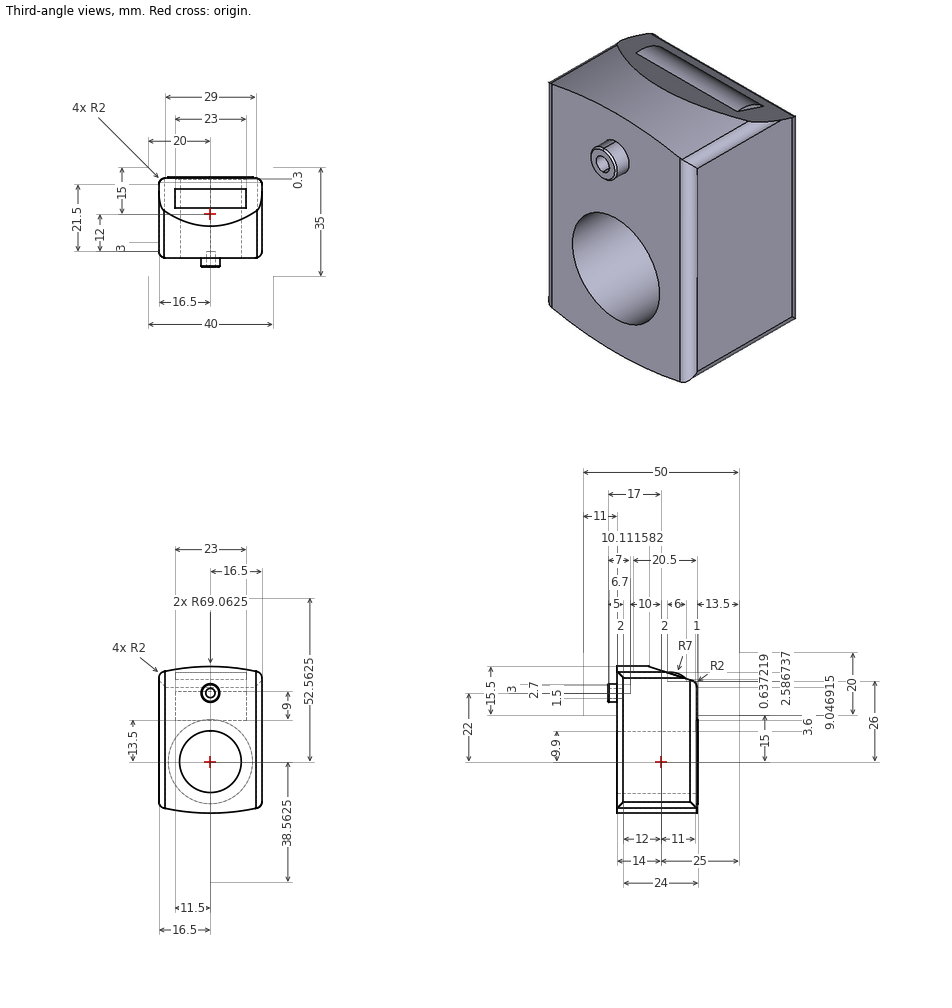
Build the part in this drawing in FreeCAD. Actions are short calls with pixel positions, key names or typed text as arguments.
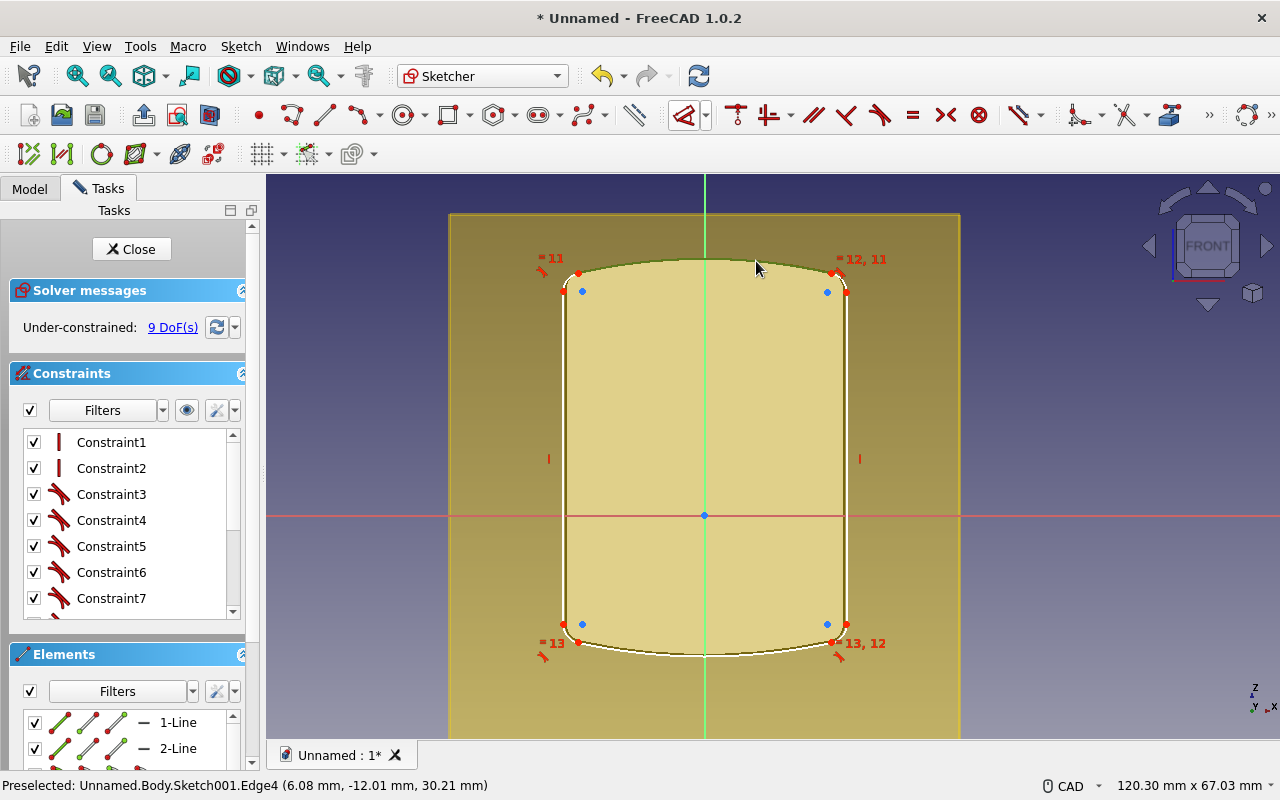
click(654, 654)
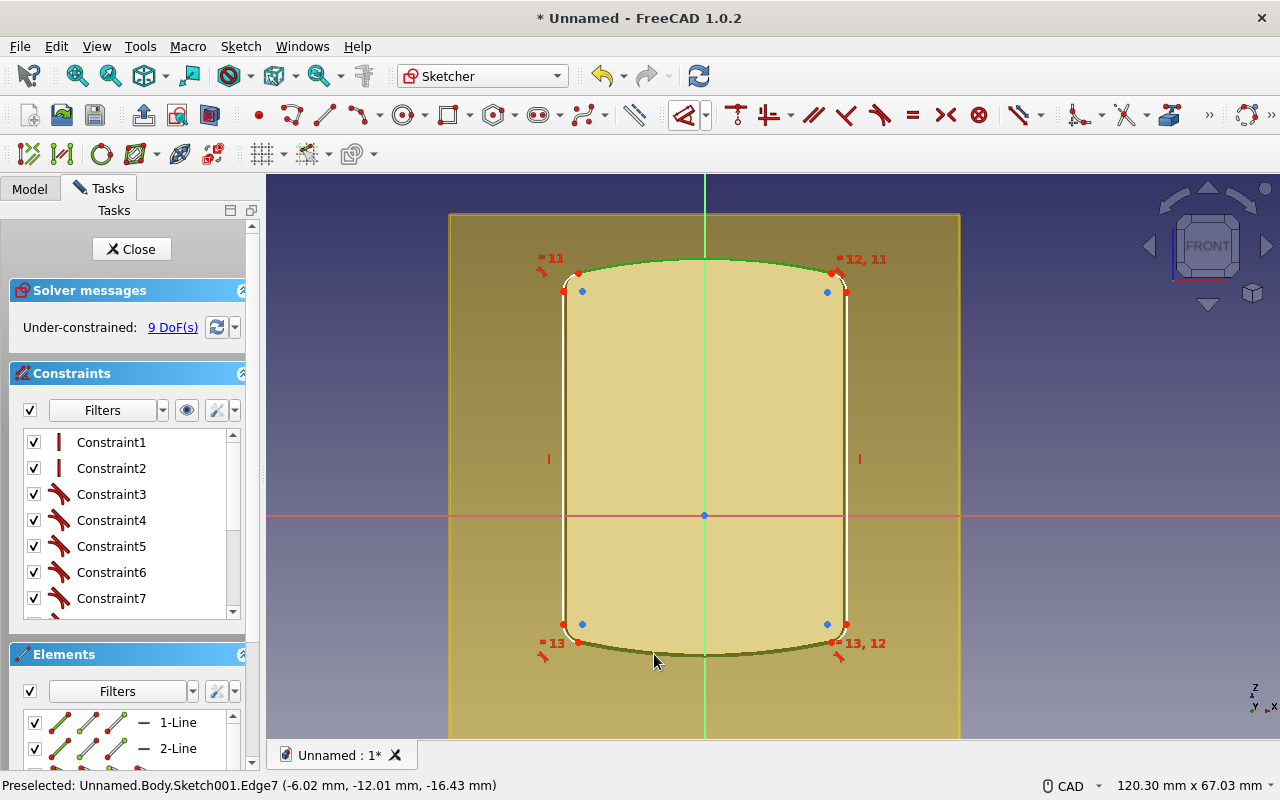
click(913, 116)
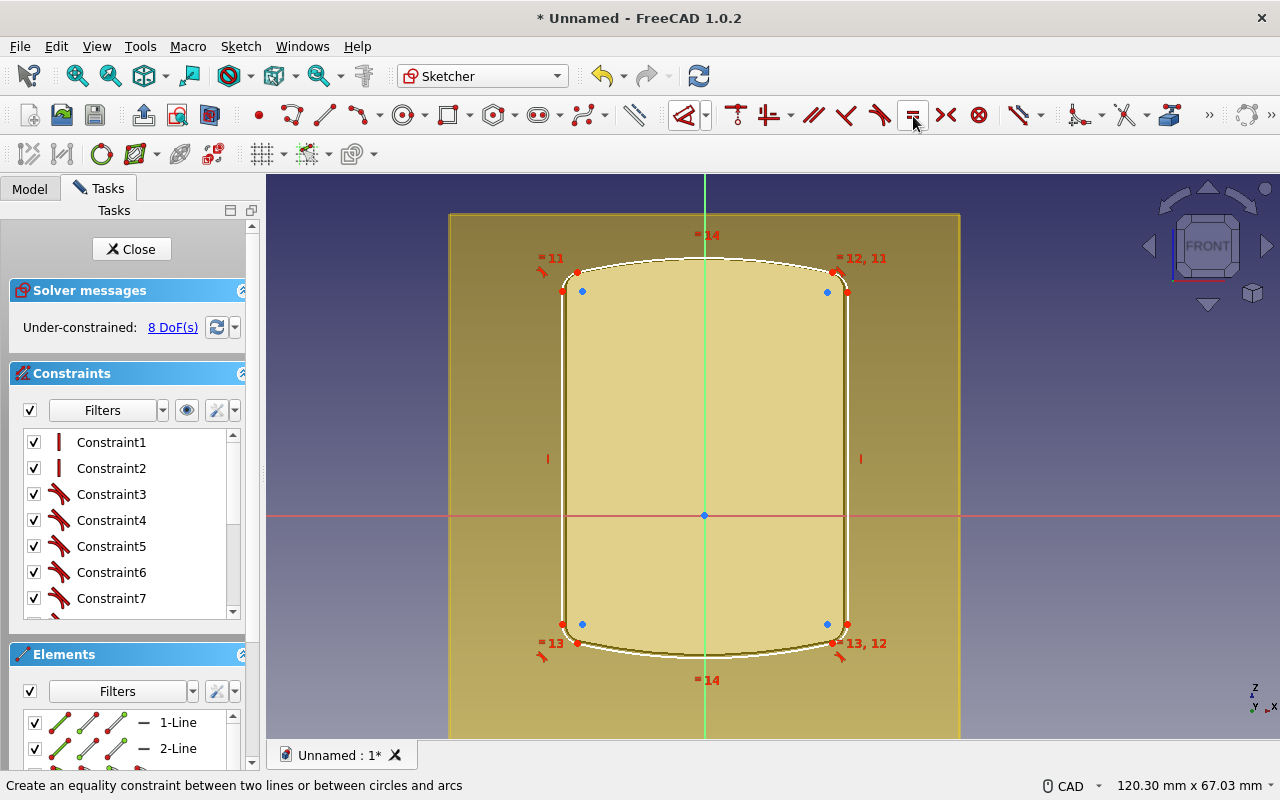
scroll(704, 283, down, 2)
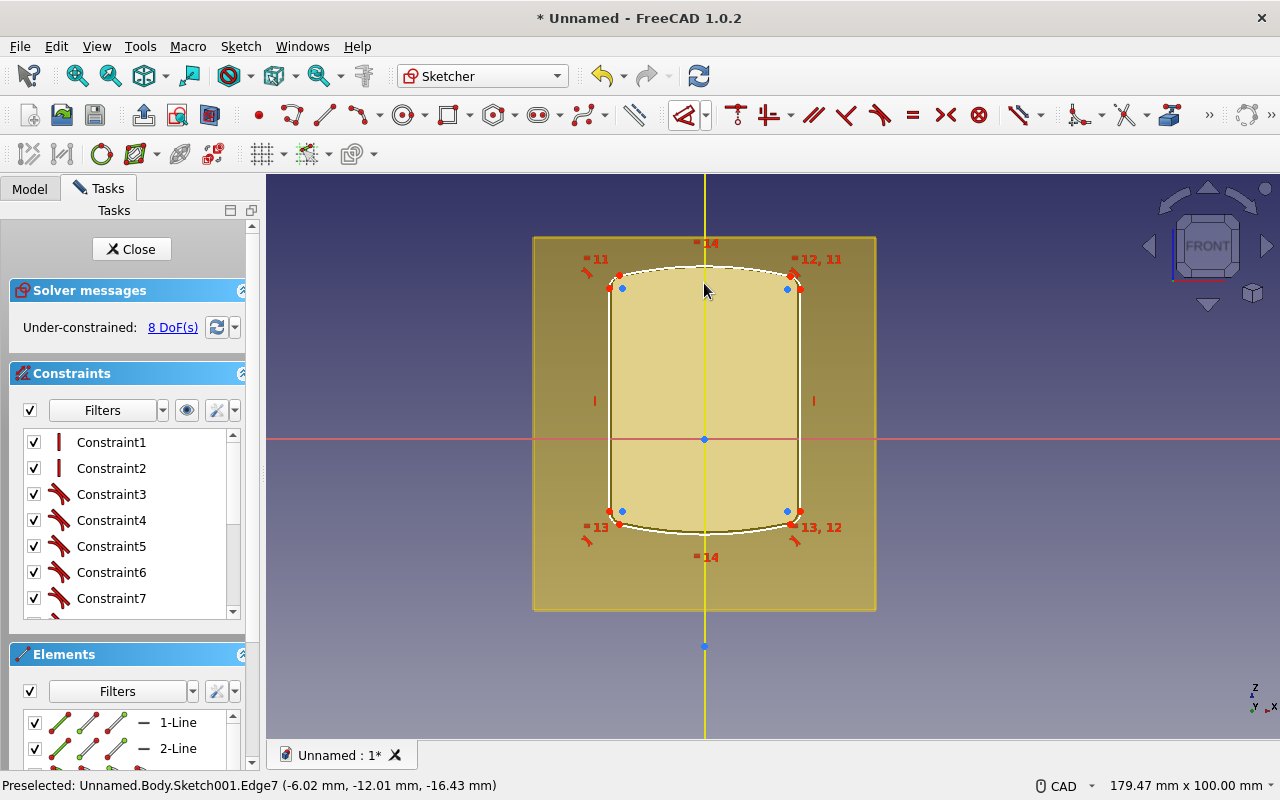
click(704, 646)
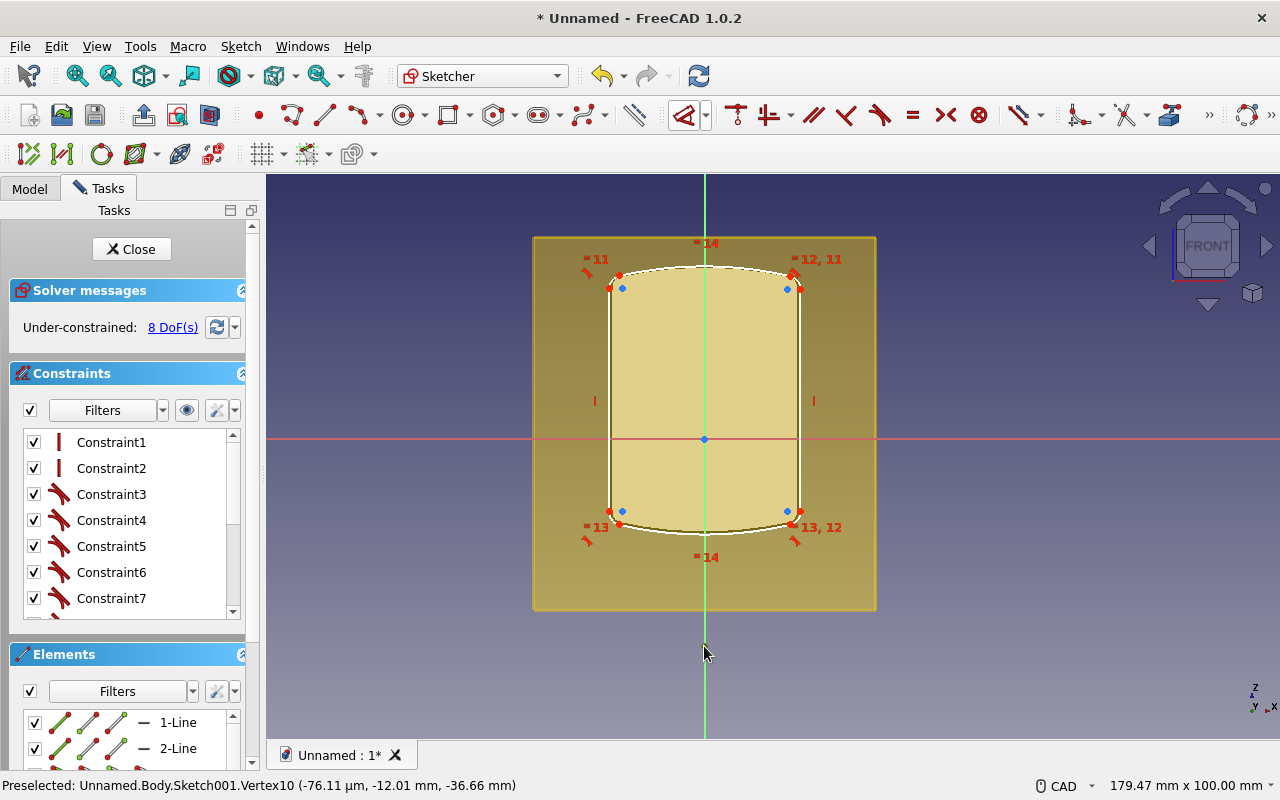
click(705, 675)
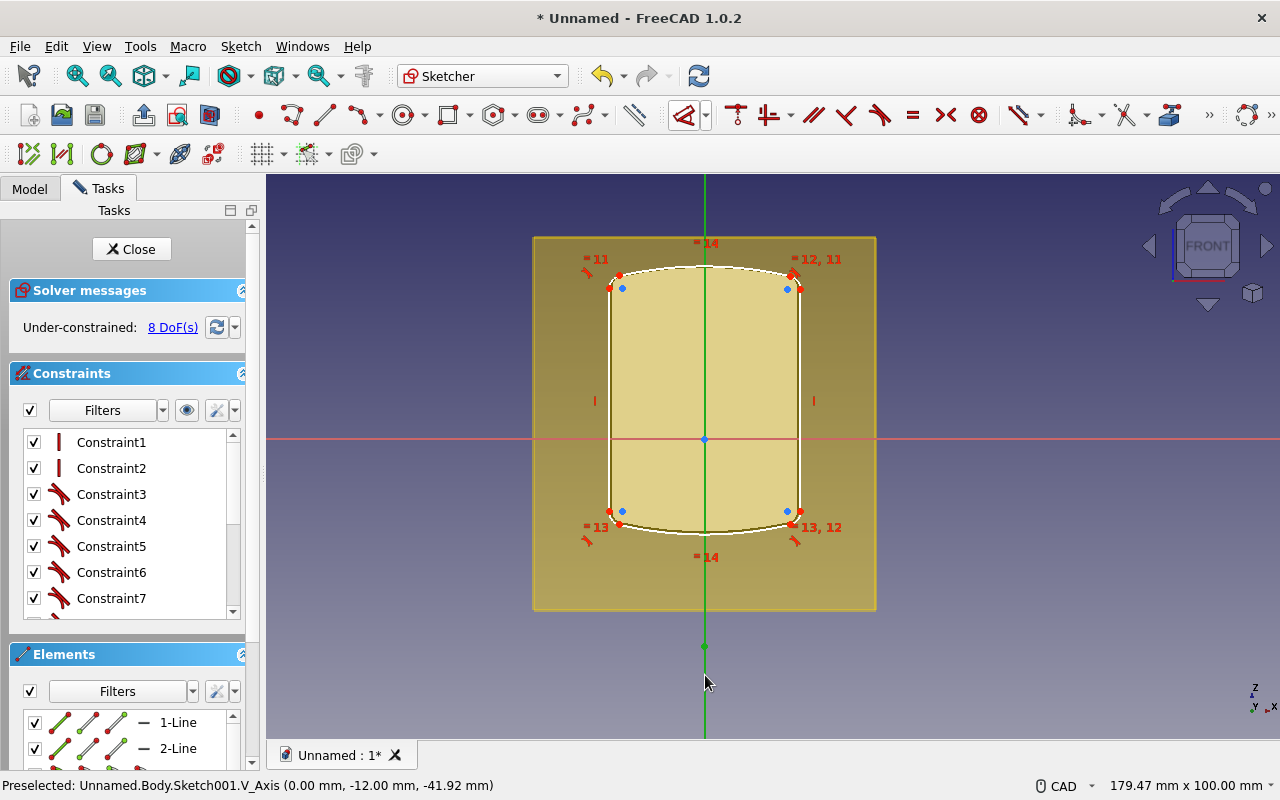
click(736, 116)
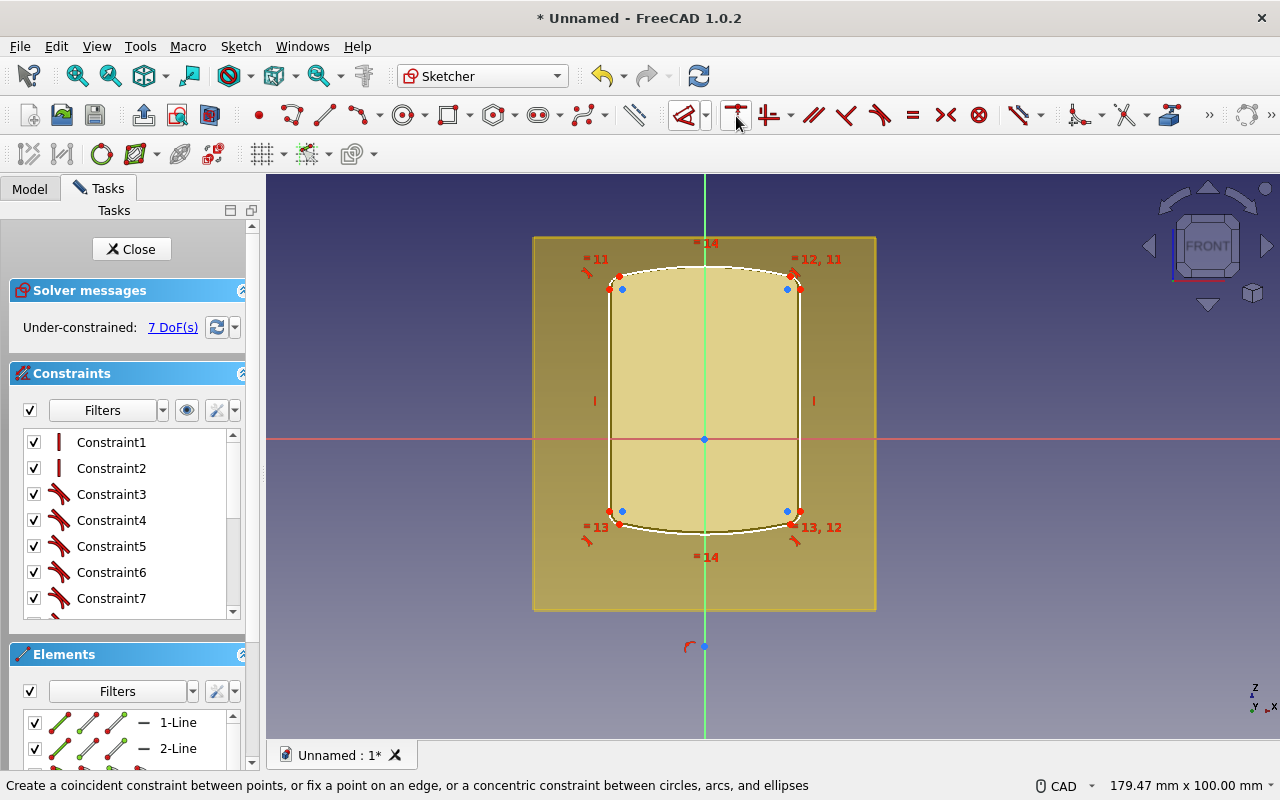
scroll(705, 284, up, 2)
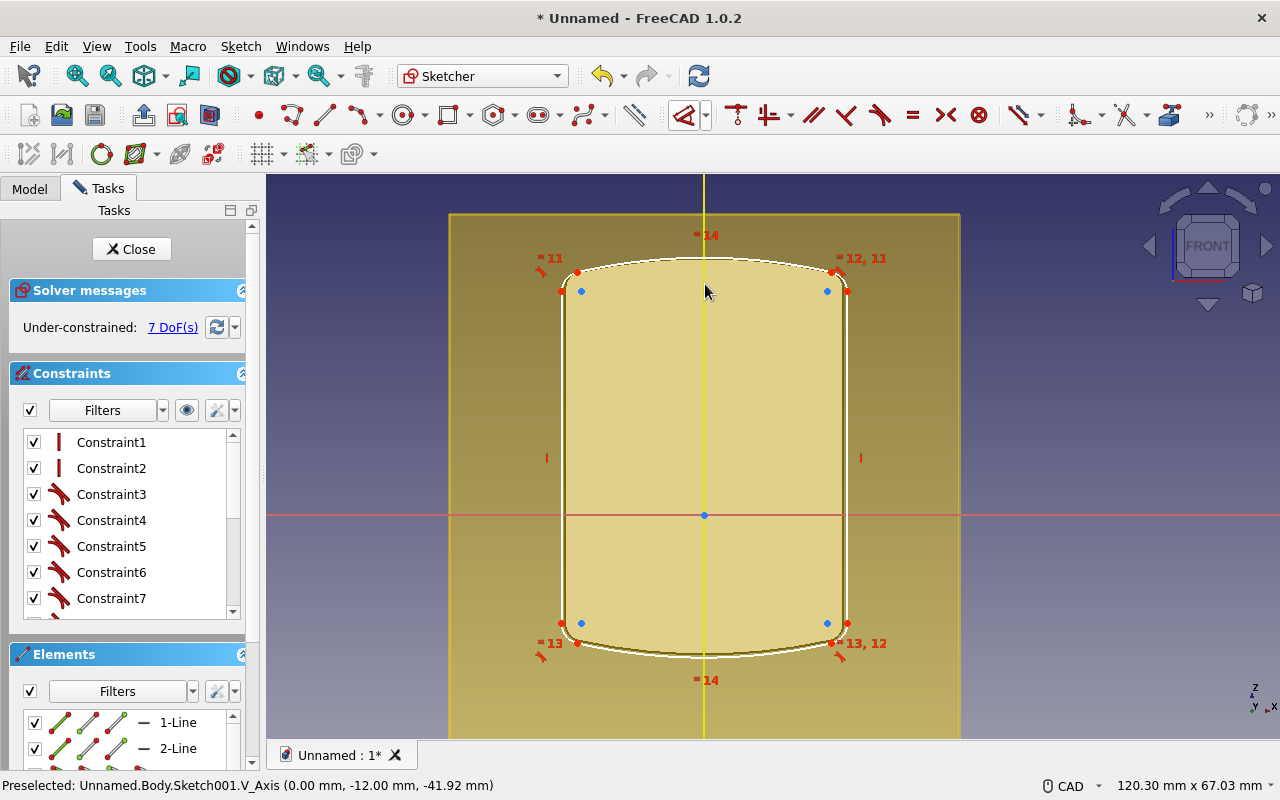
scroll(705, 627, down, 2)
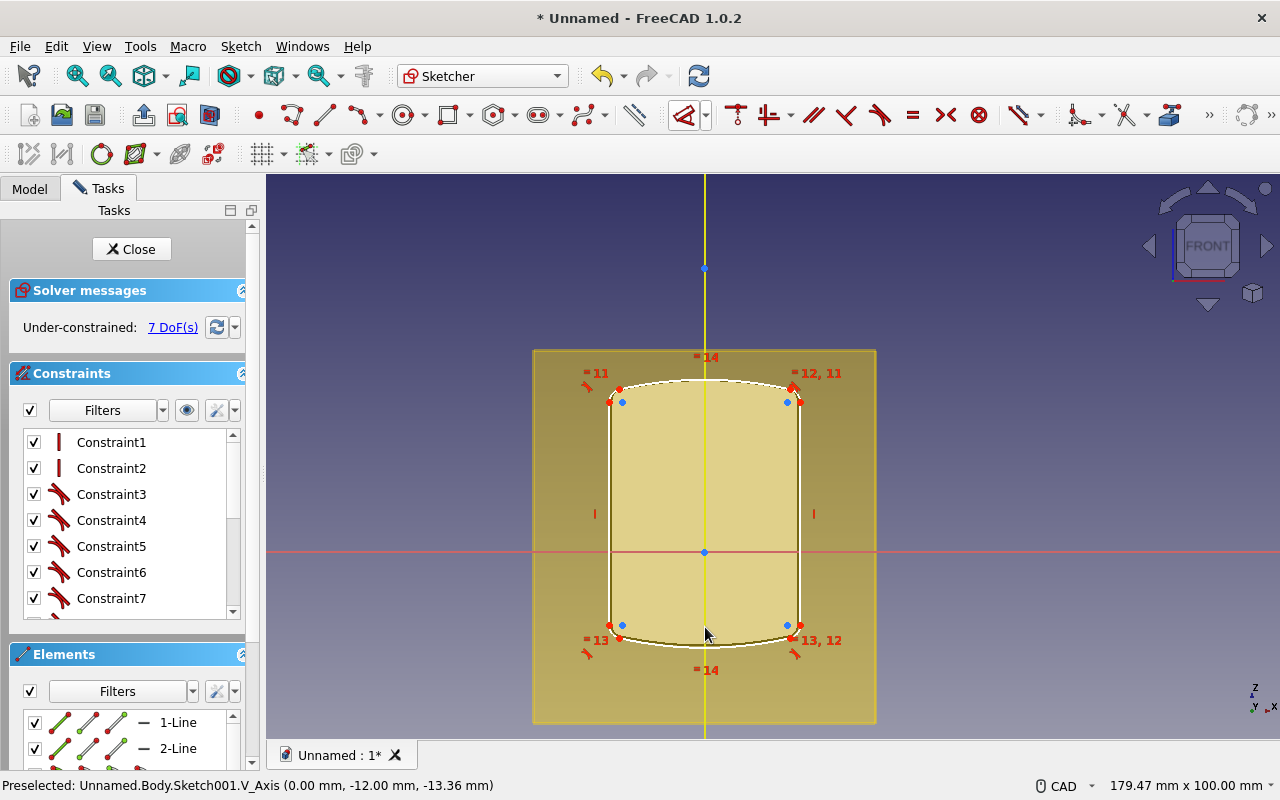
click(705, 268)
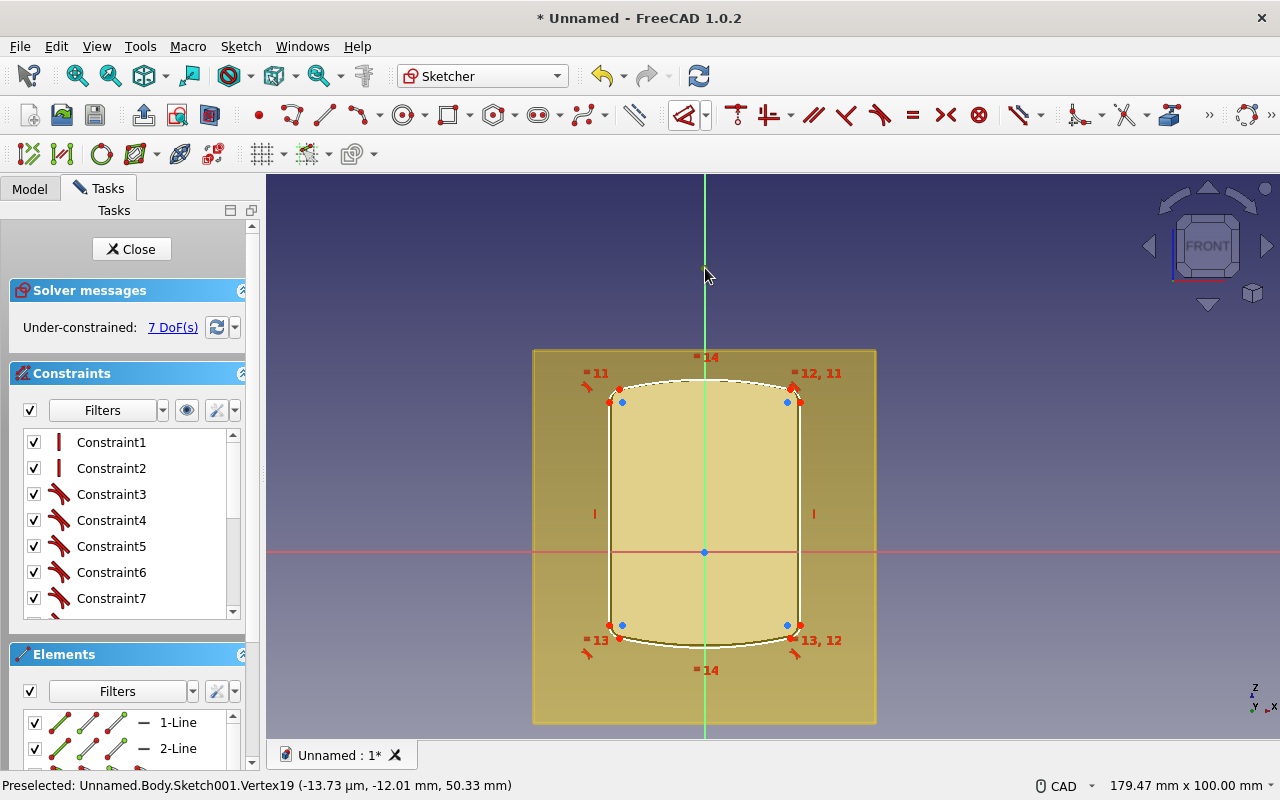
click(705, 602)